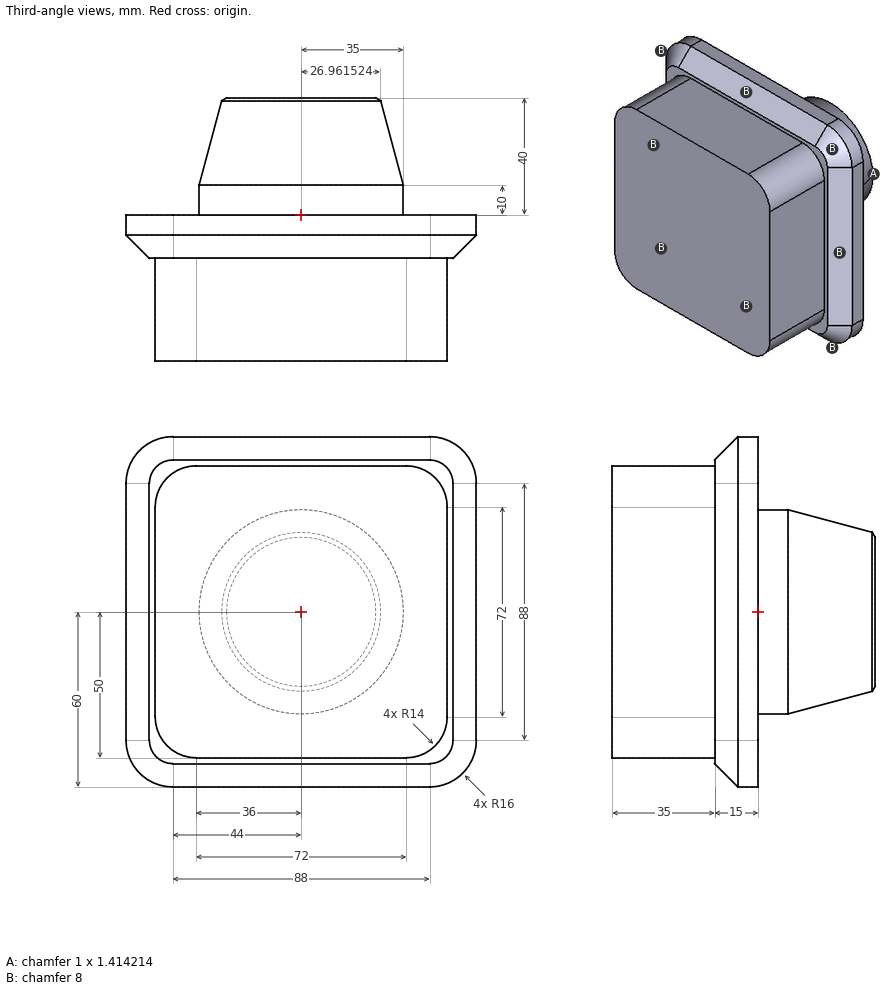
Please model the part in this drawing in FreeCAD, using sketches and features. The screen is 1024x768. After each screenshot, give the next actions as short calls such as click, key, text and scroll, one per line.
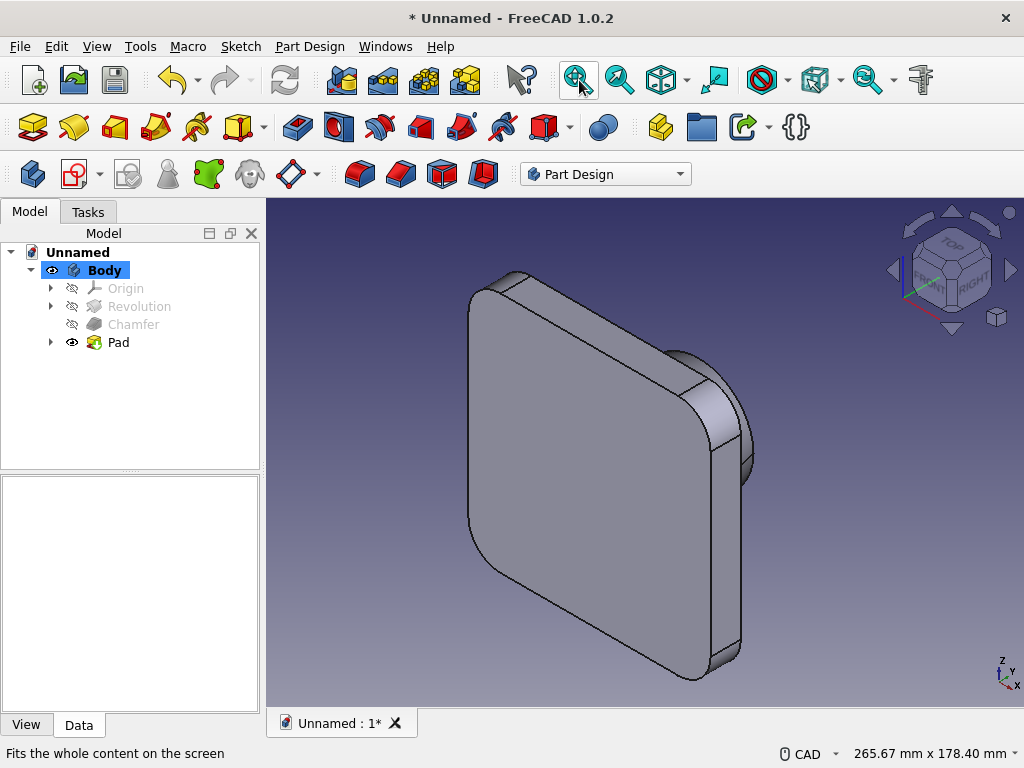
click(590, 484)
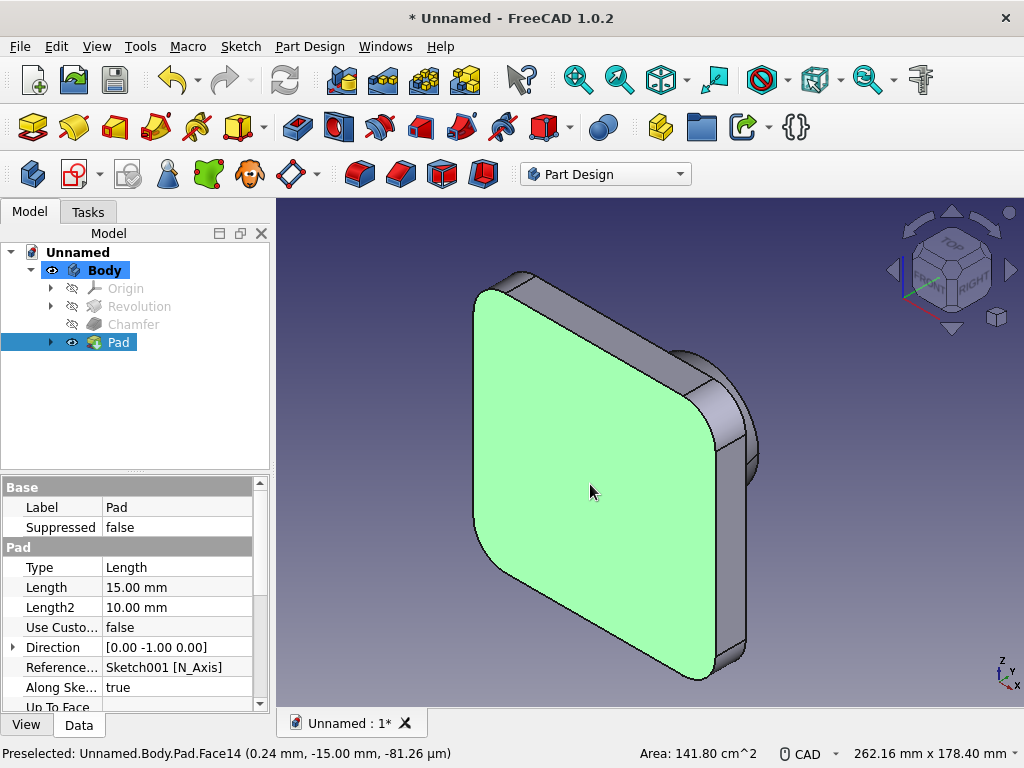
click(74, 174)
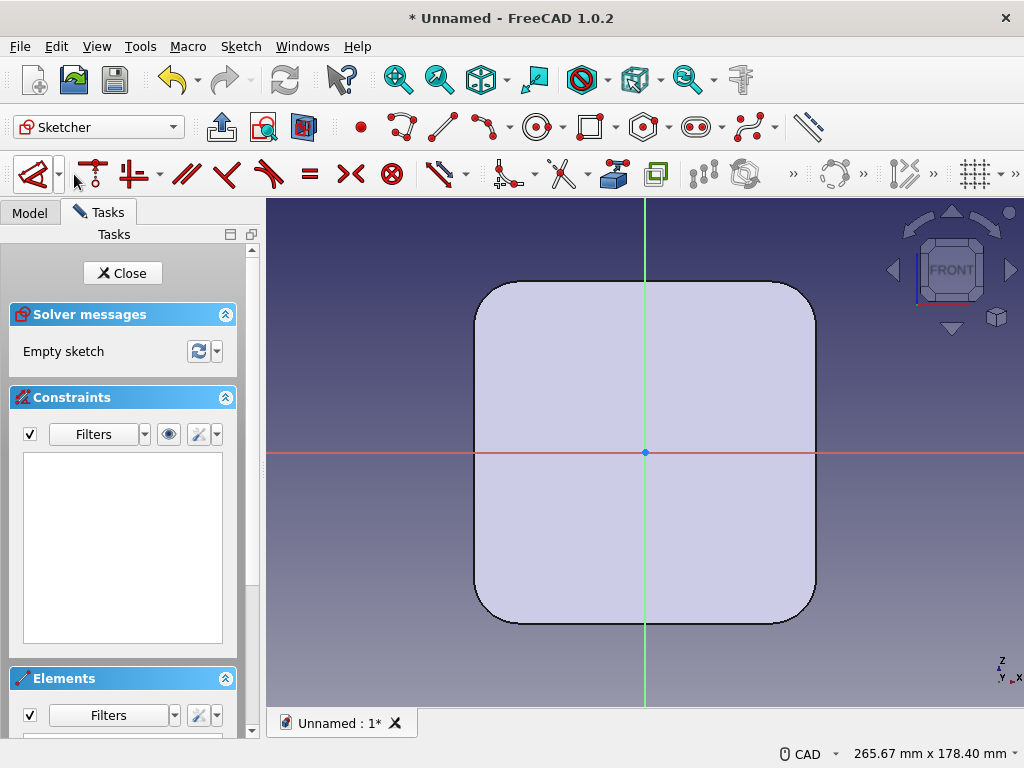
key(g)
key(l)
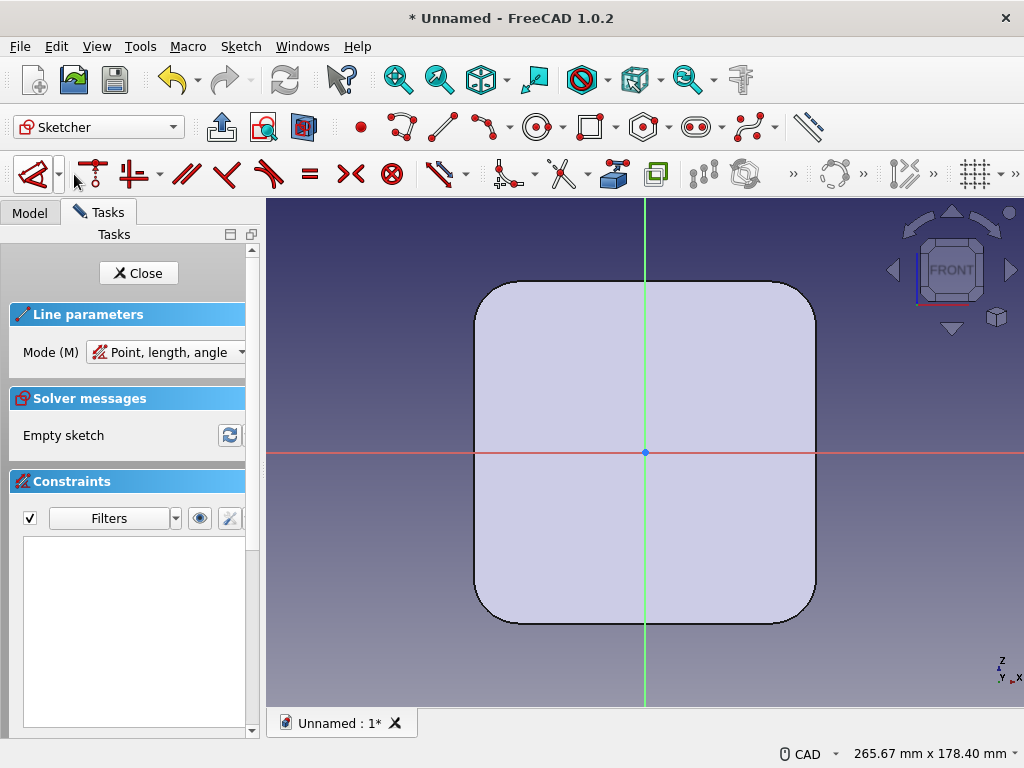
click(542, 595)
click(748, 595)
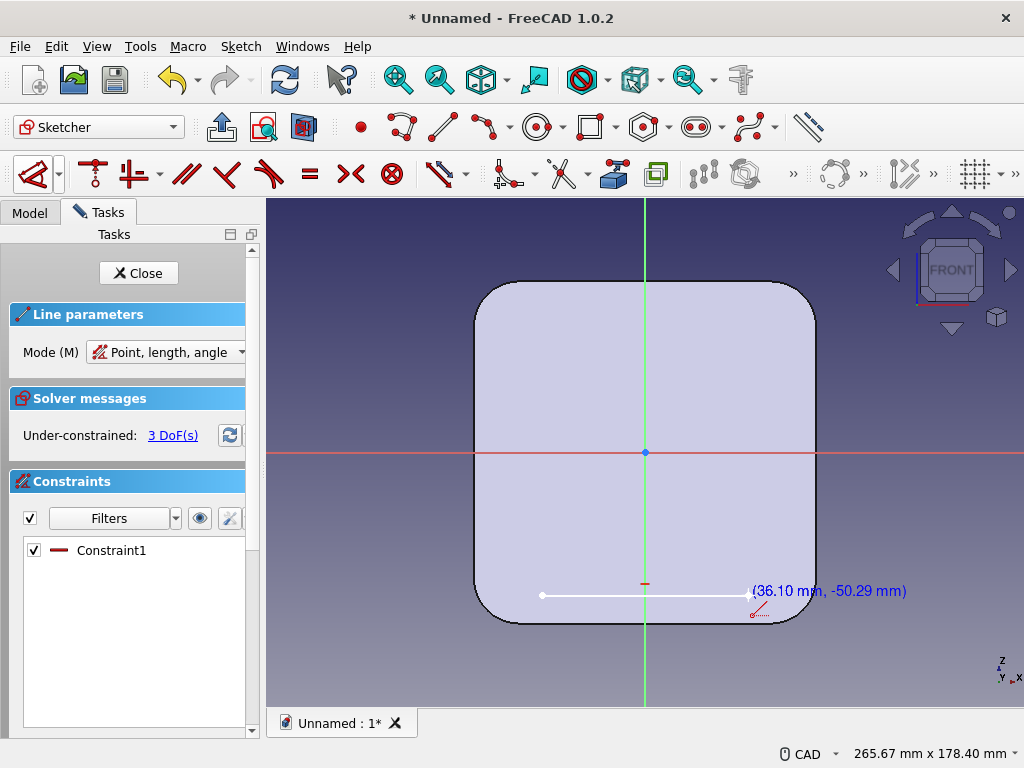
click(788, 555)
click(788, 350)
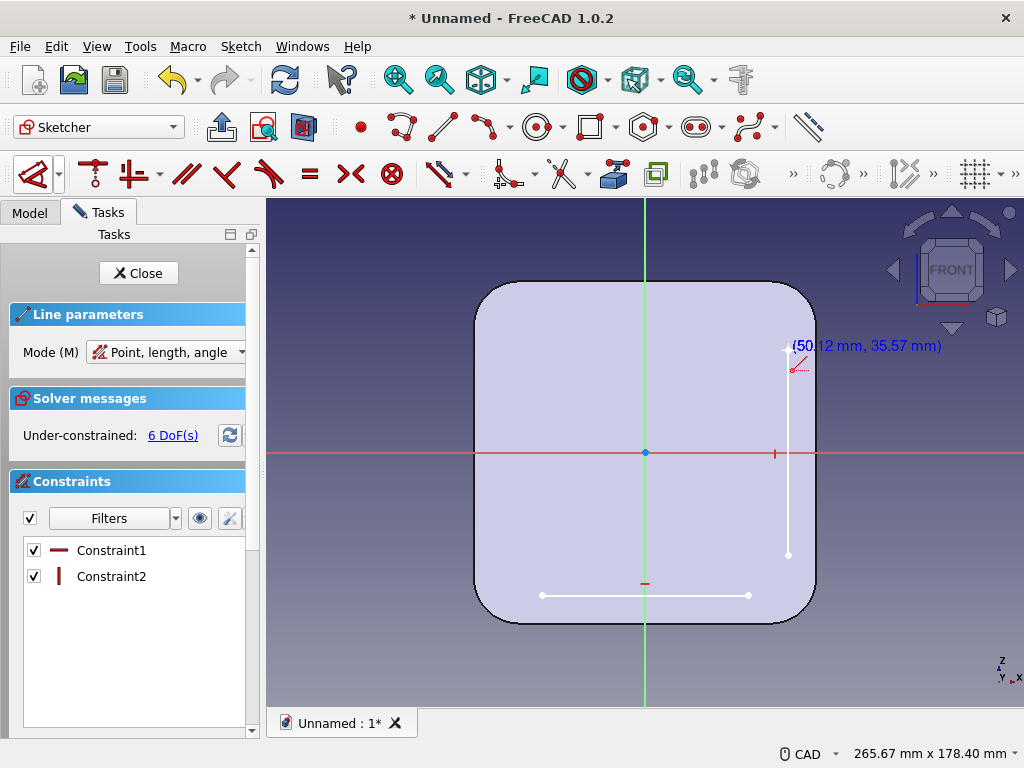
click(748, 310)
click(542, 310)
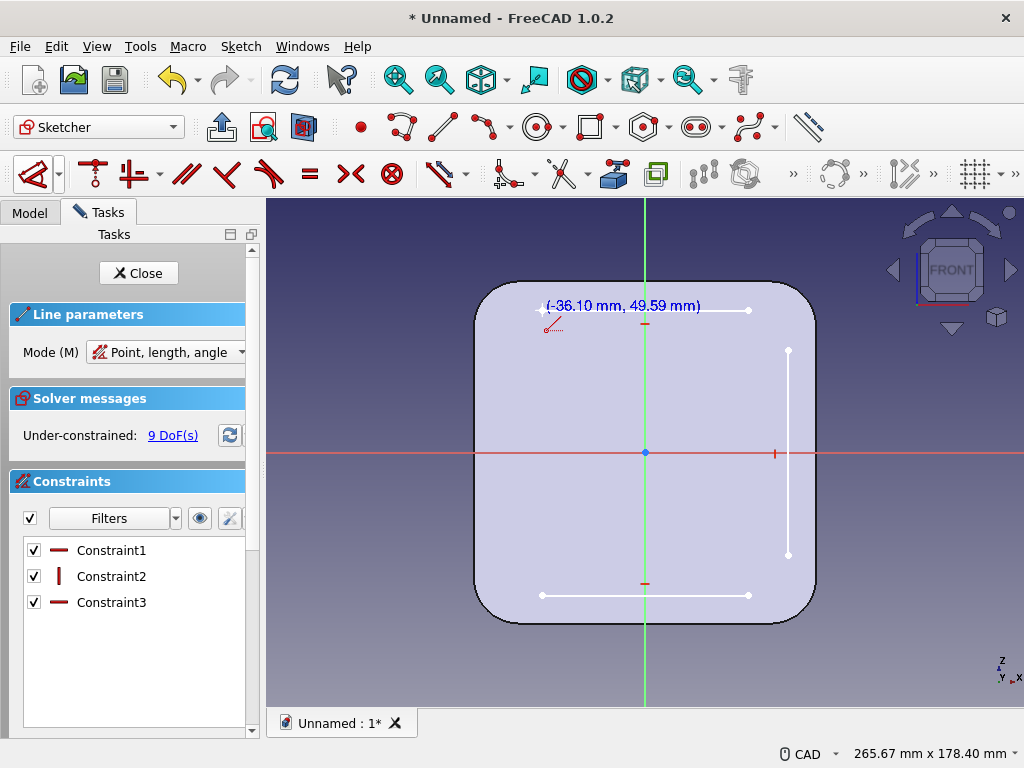
click(502, 350)
click(502, 555)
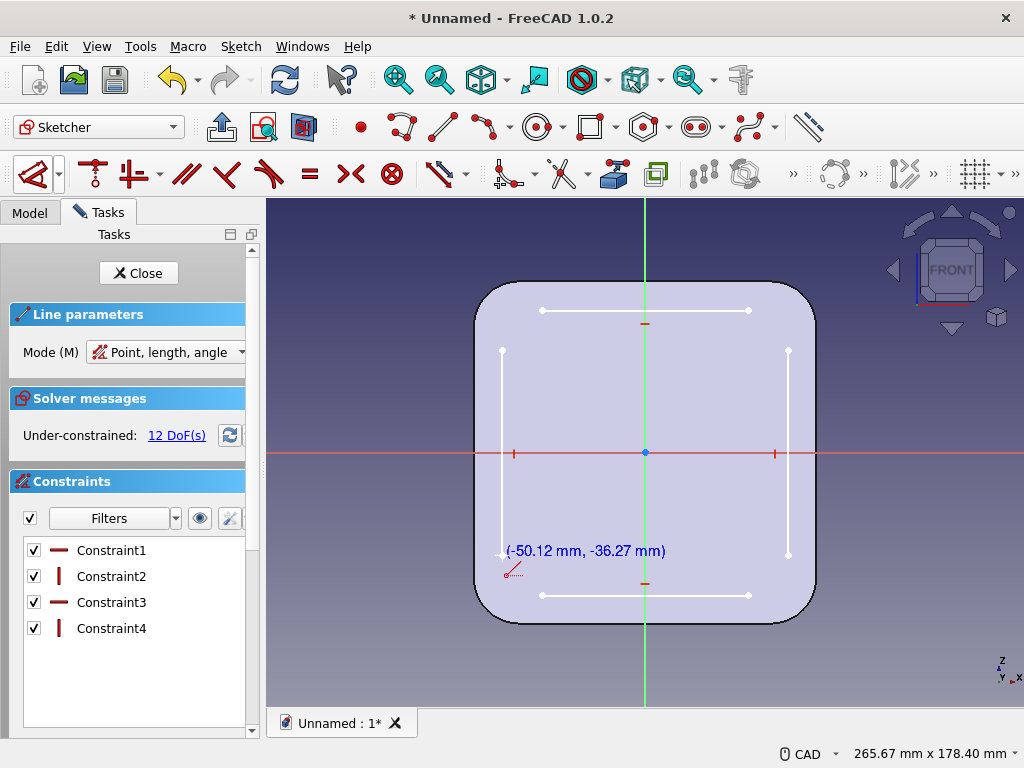
key(g)
key(3)
key(a)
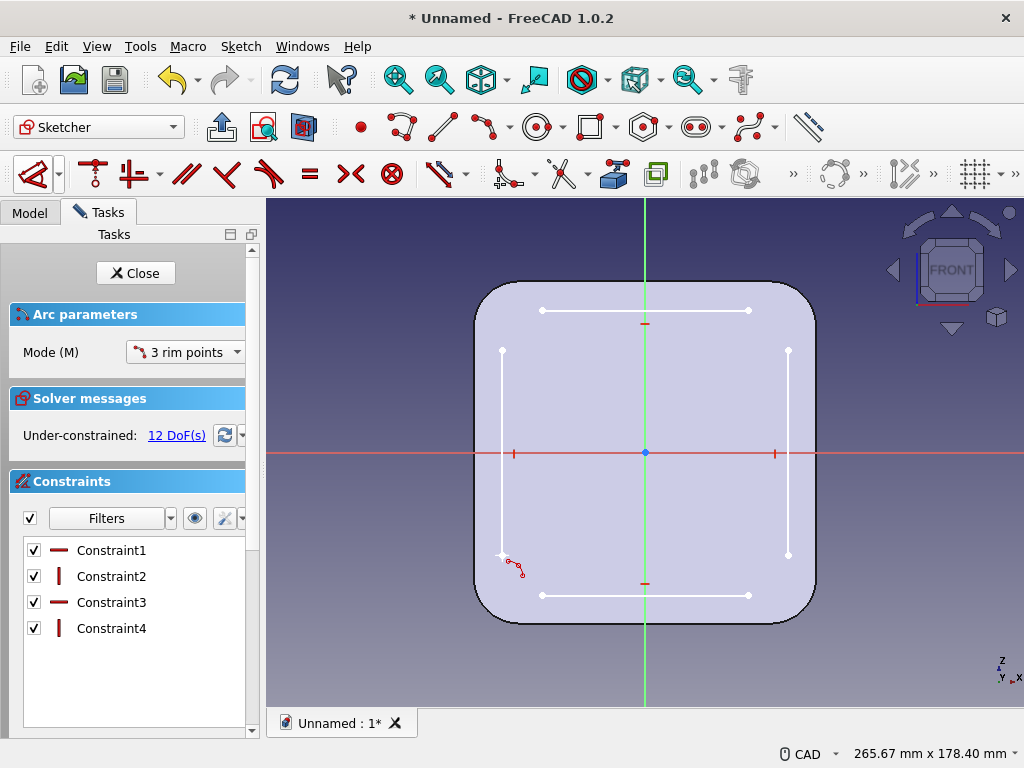
click(748, 596)
click(788, 556)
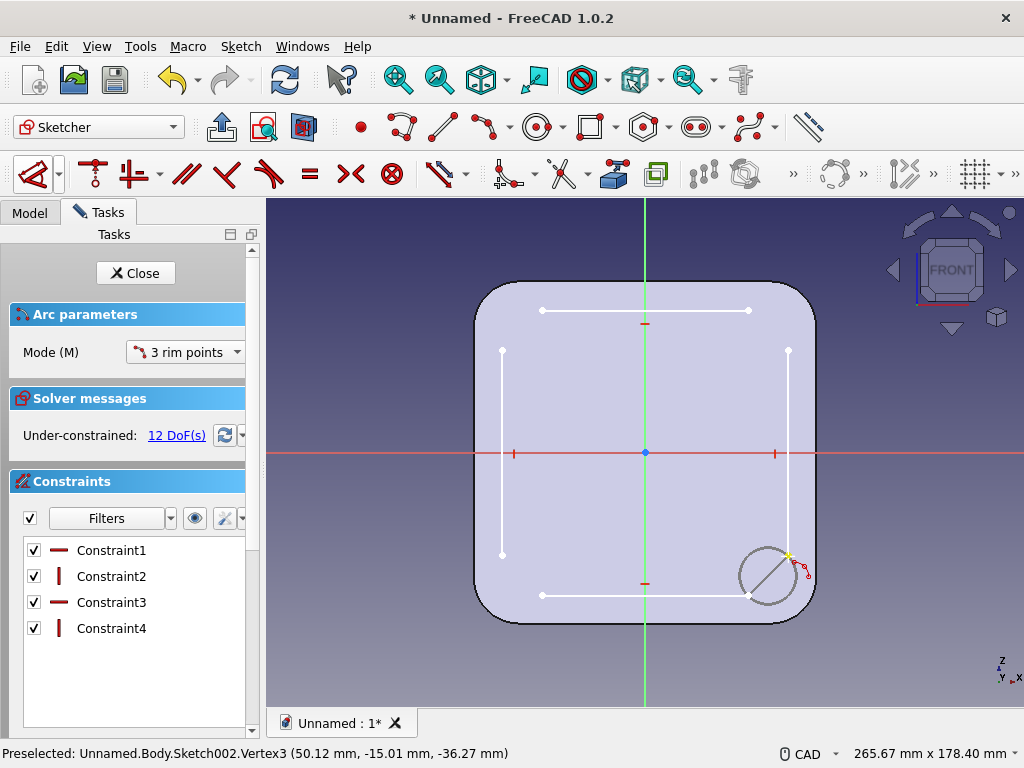
scroll(776, 583, up, 2)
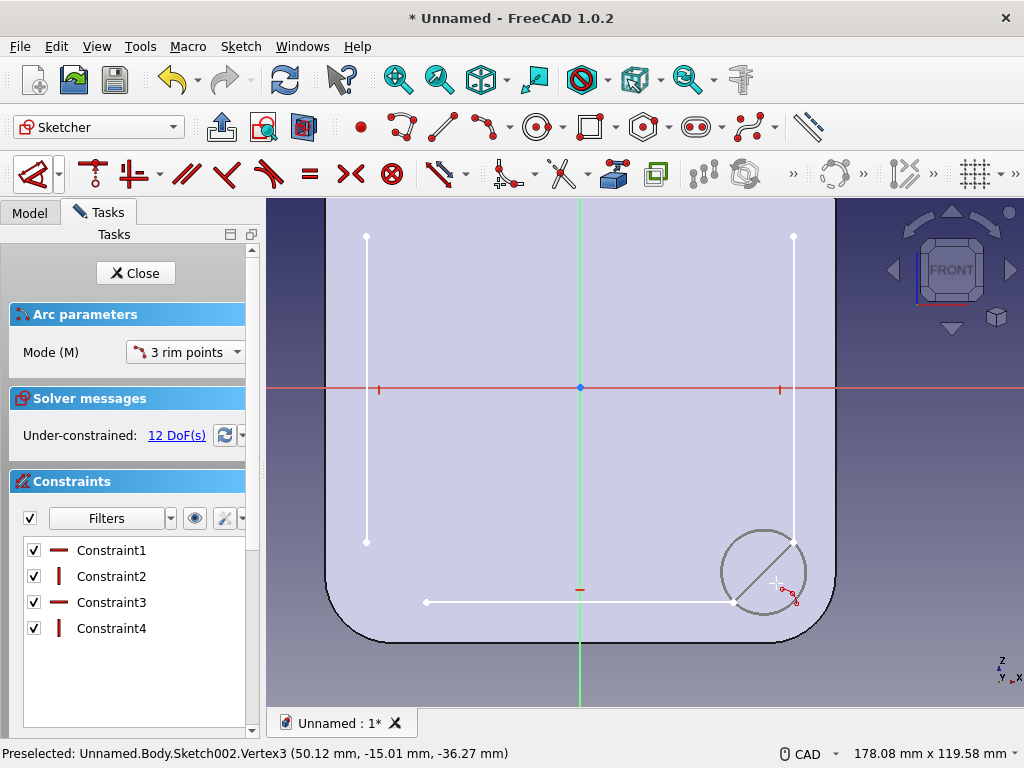
click(776, 583)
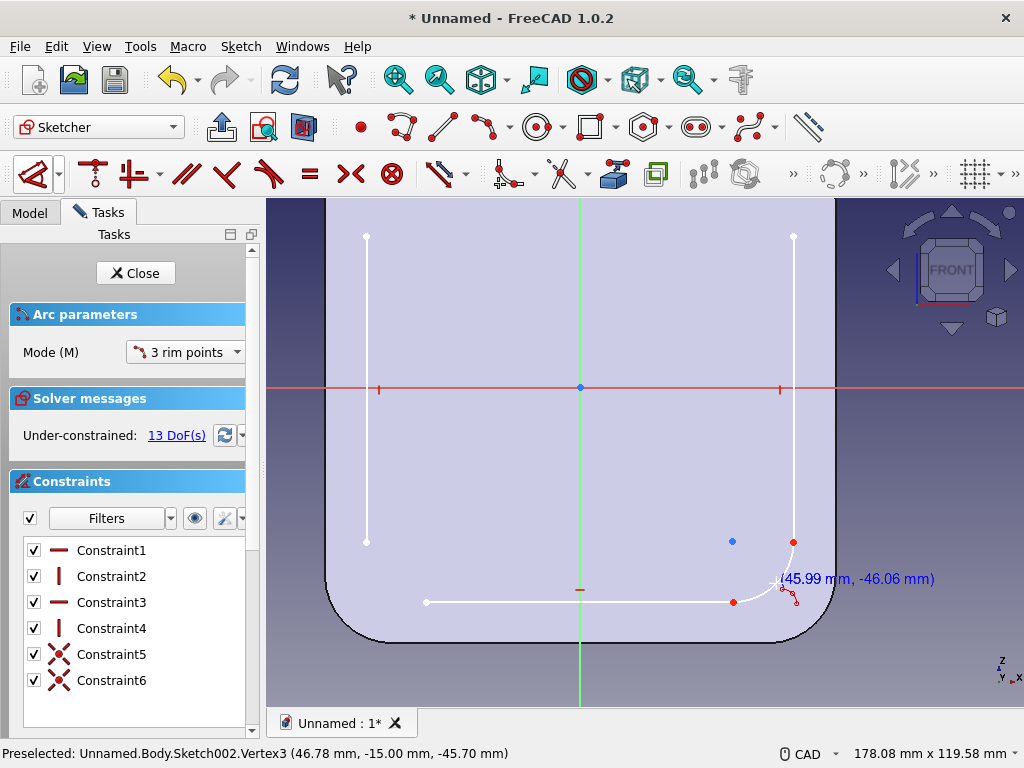
click(794, 237)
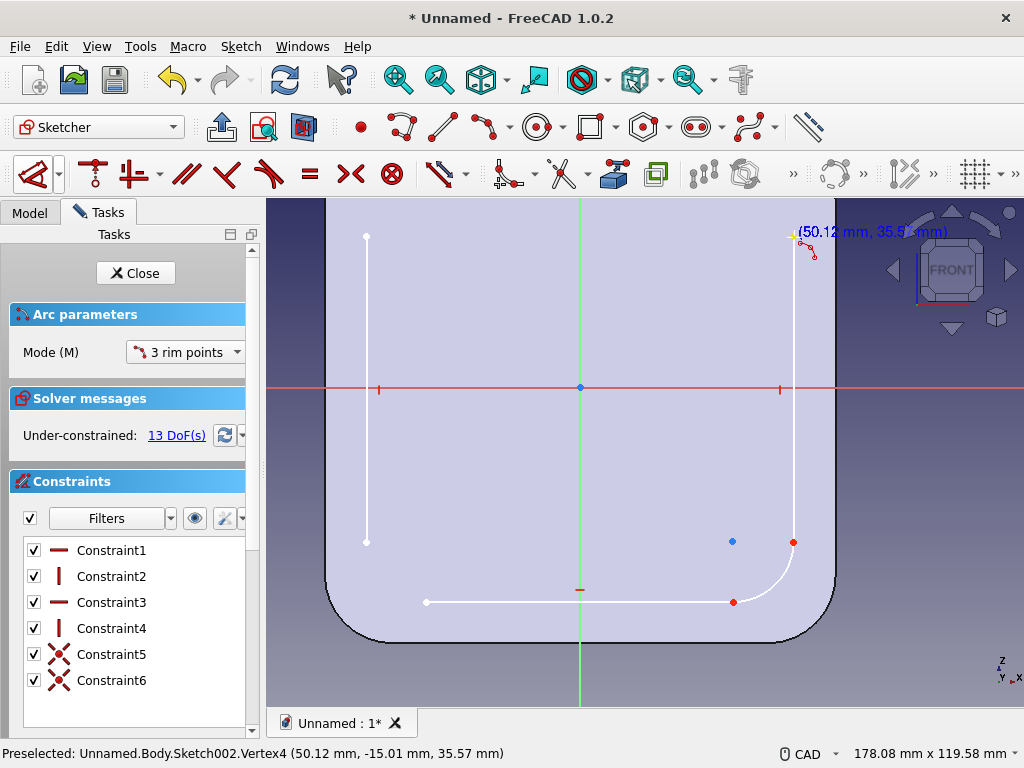
scroll(560, 679, down, 1)